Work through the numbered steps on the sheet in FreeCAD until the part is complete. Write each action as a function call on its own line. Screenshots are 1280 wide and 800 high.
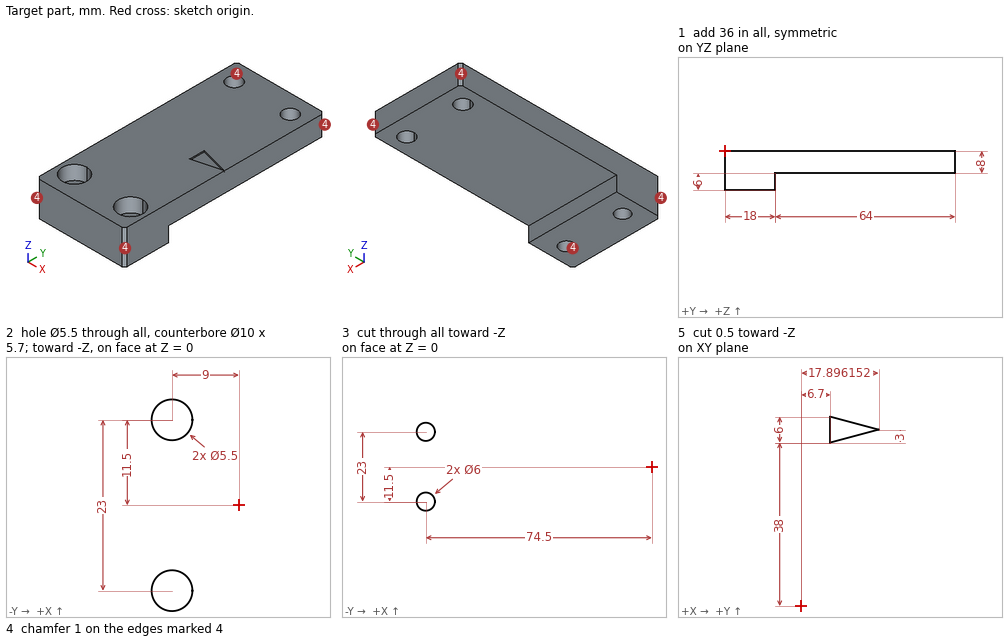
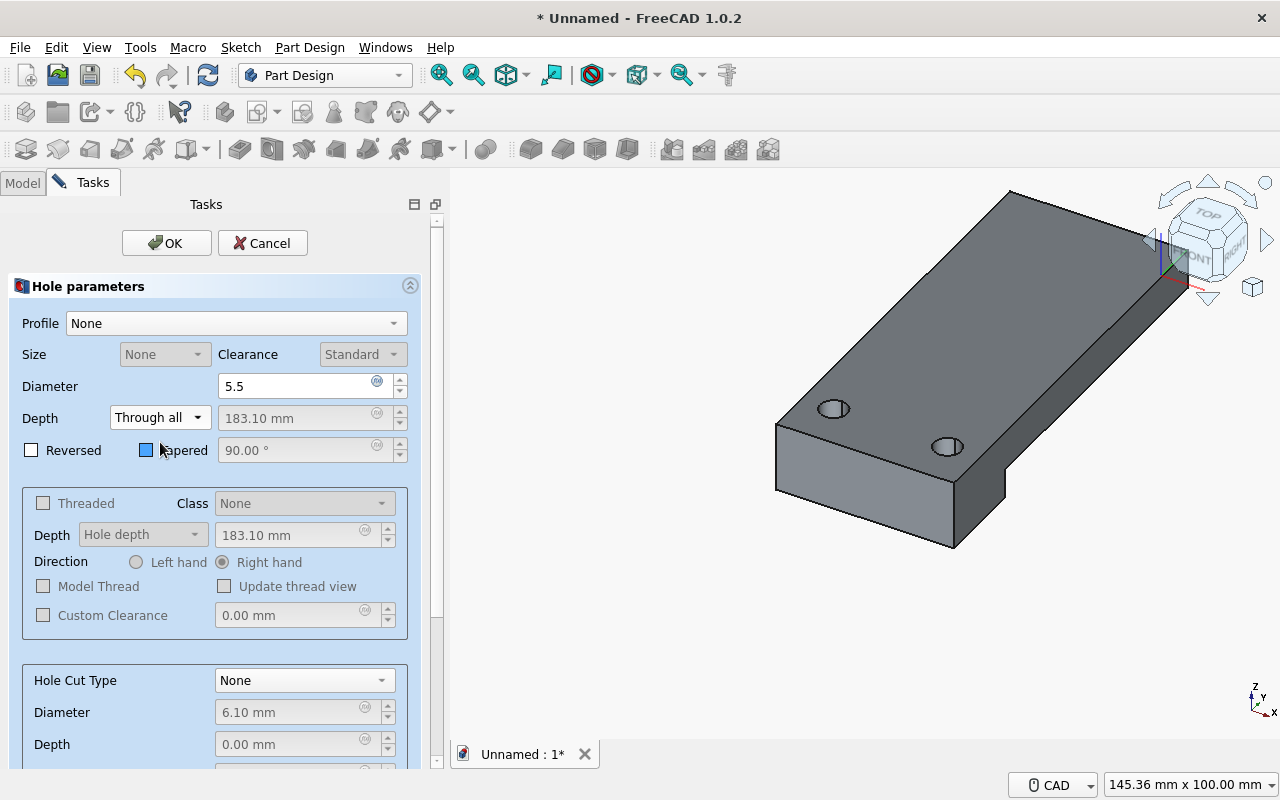
click(306, 680)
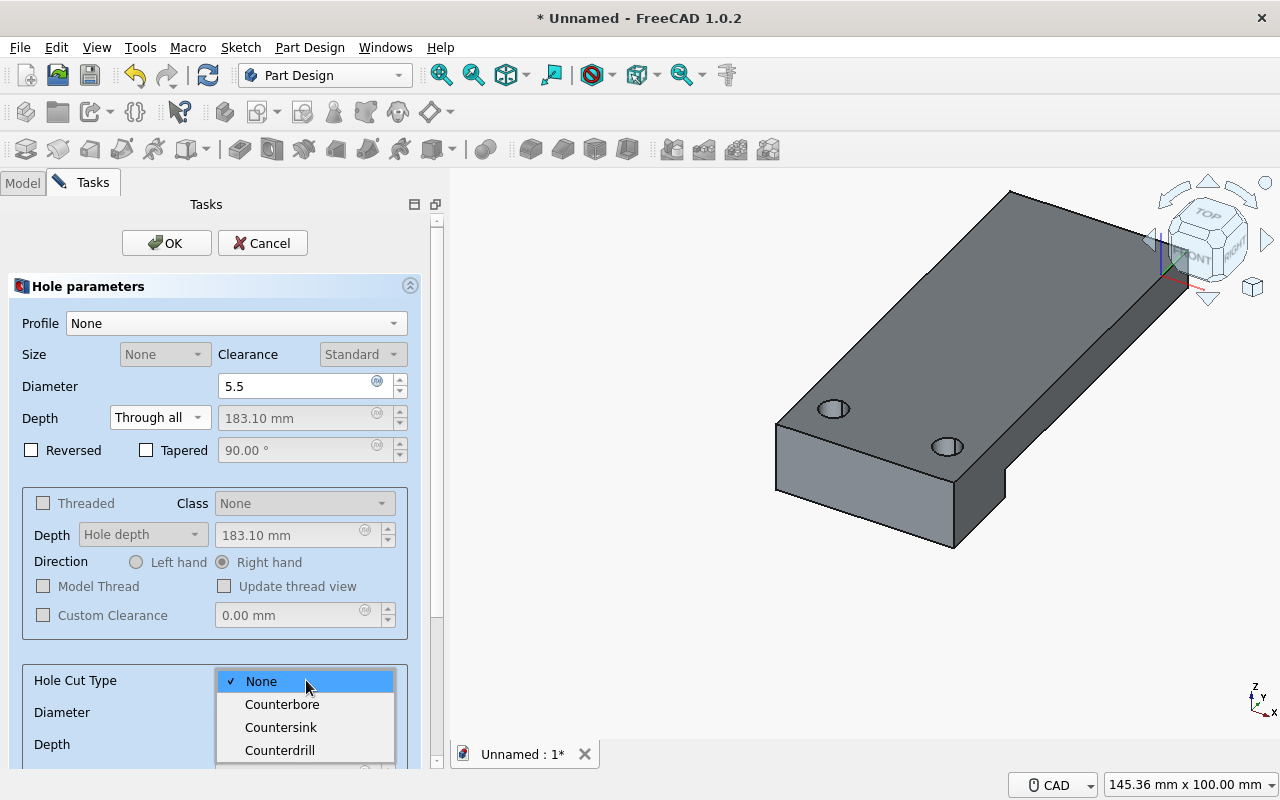
click(304, 704)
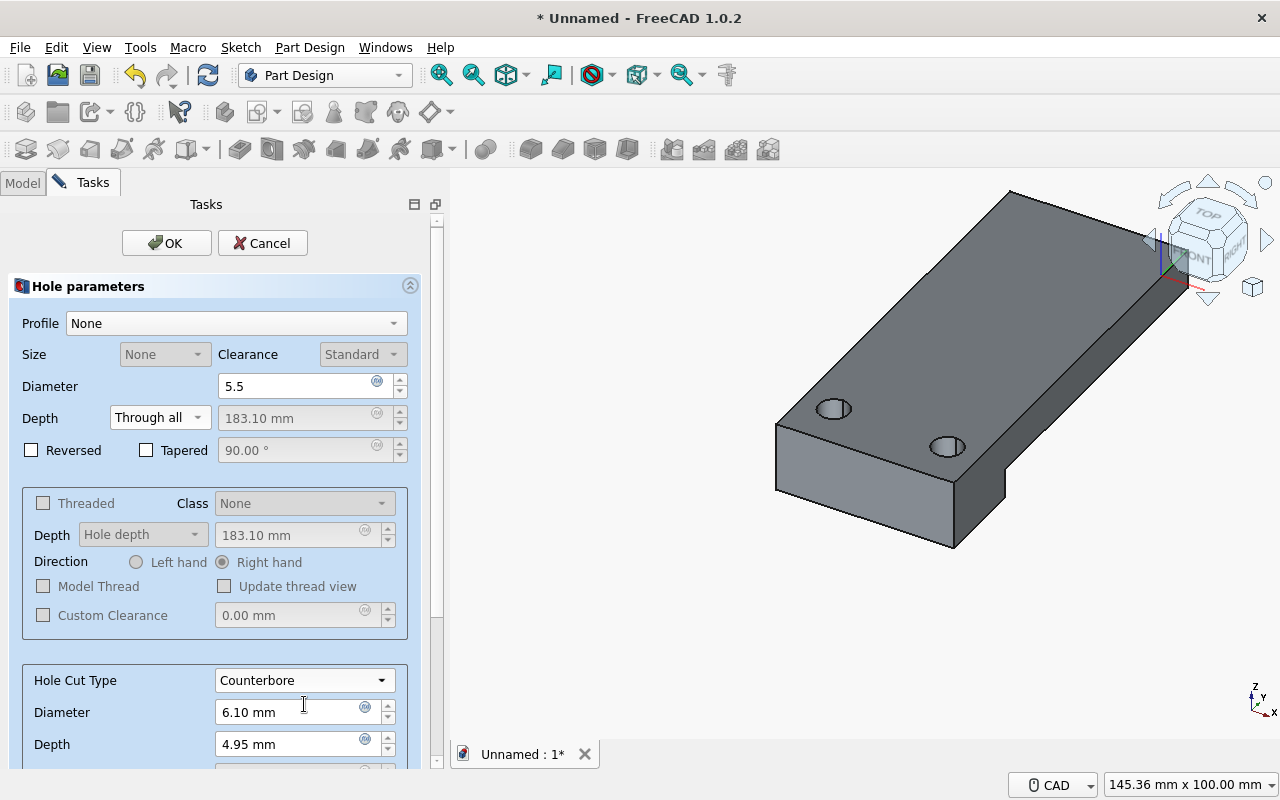
triple_click(298, 712)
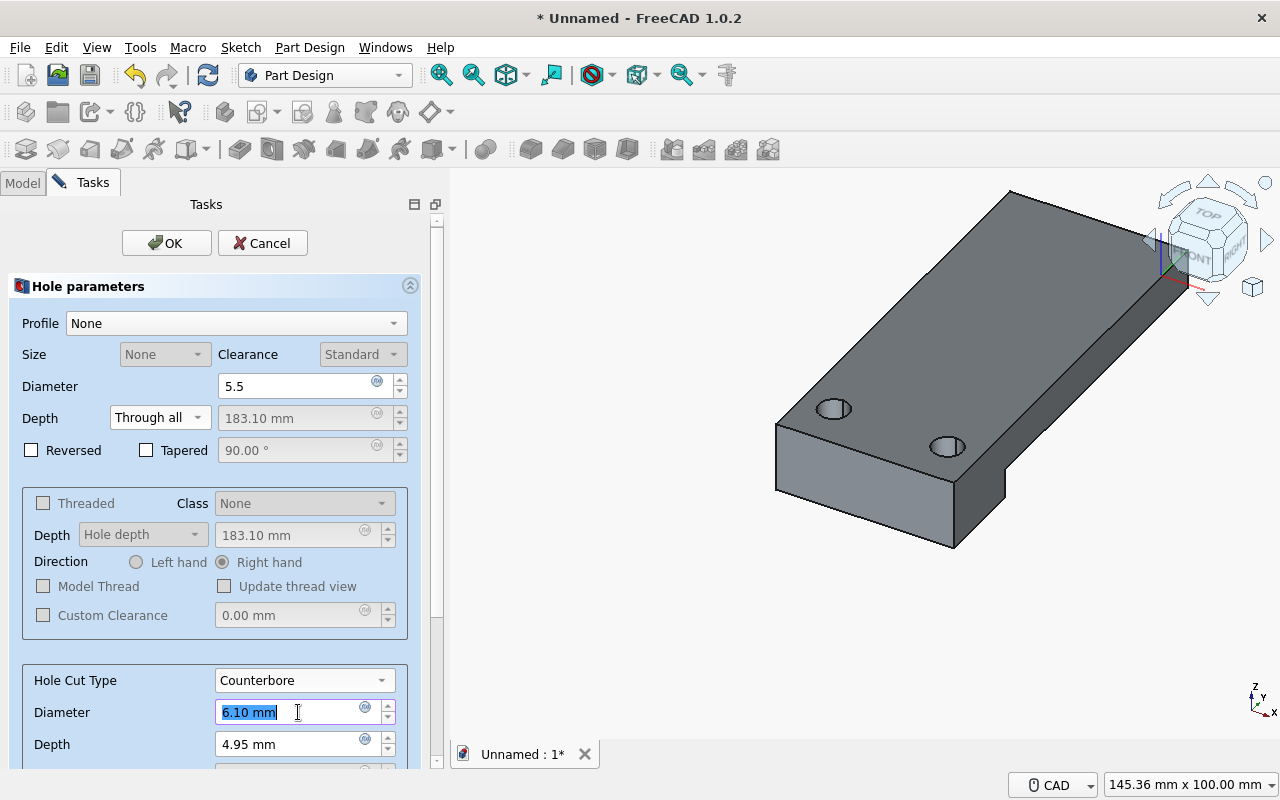
text(10)
key(Tab)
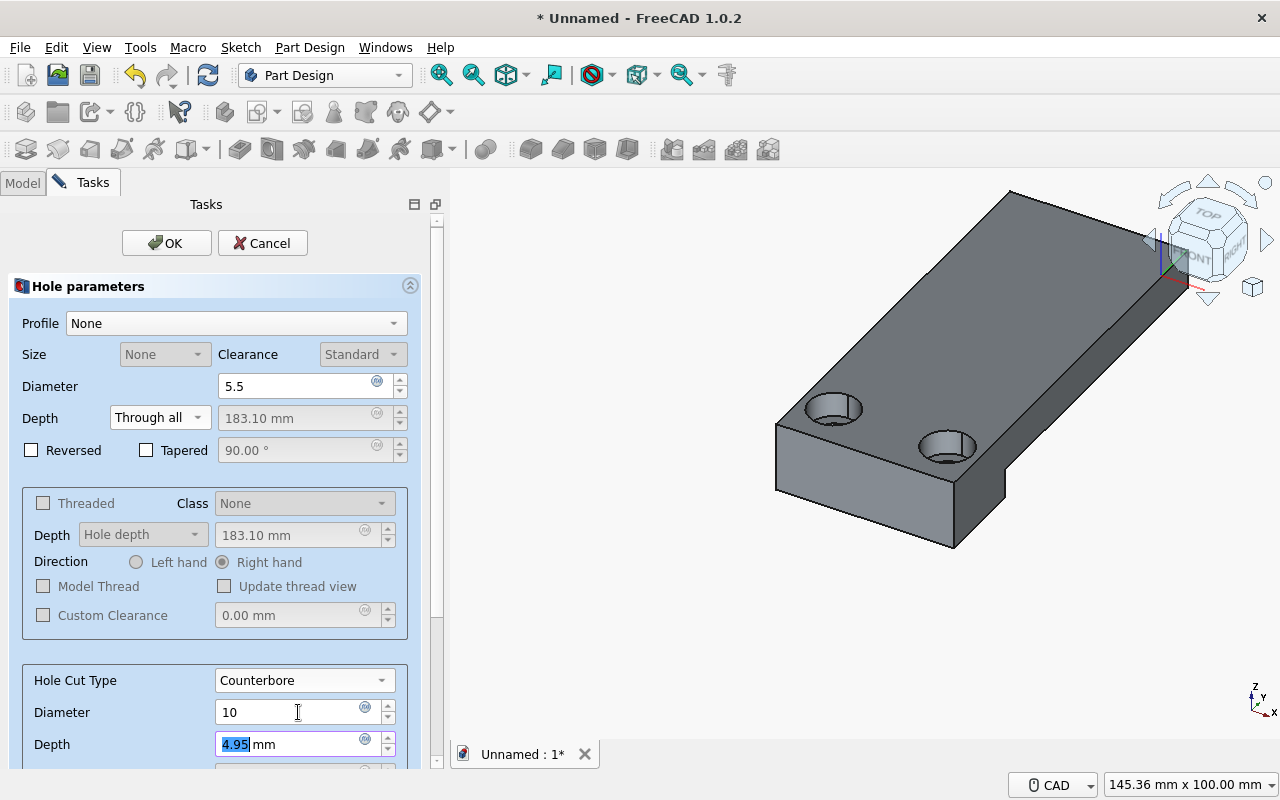
text(5.7)
key(Tab)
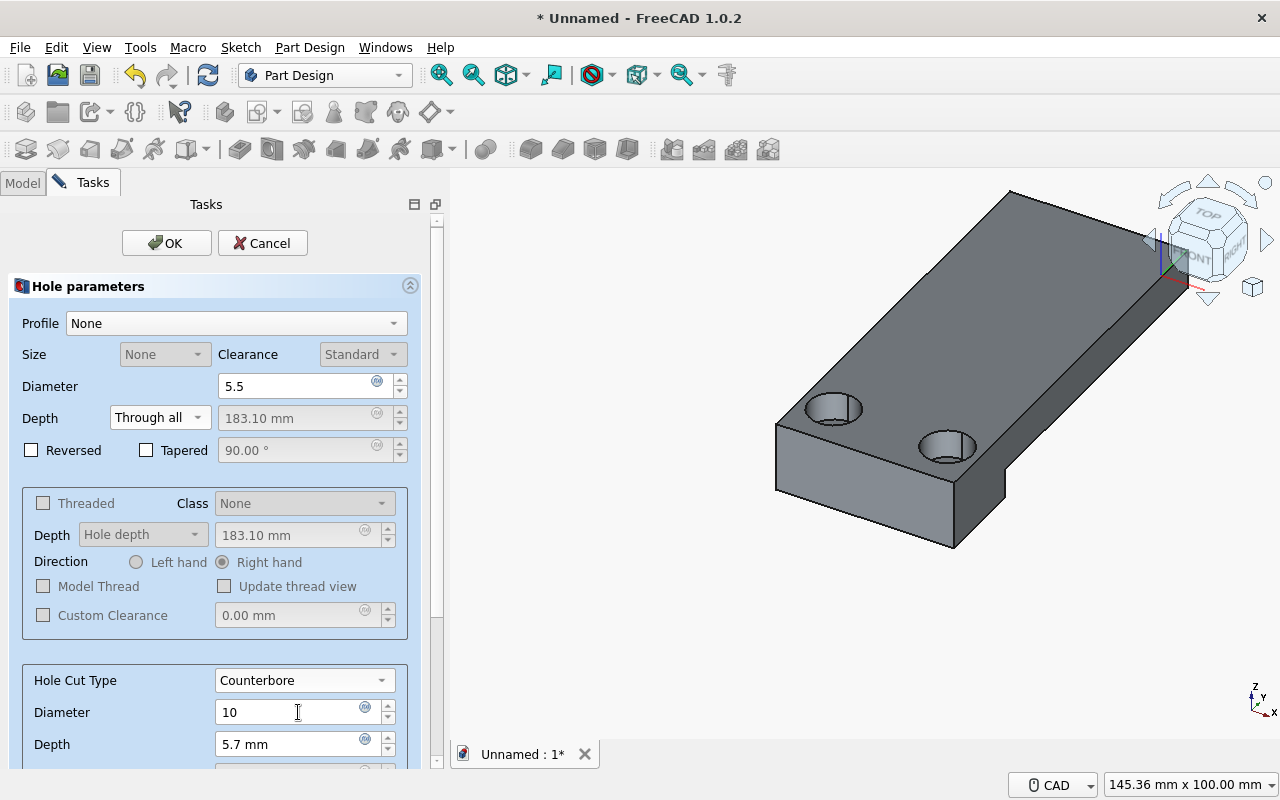
click(167, 243)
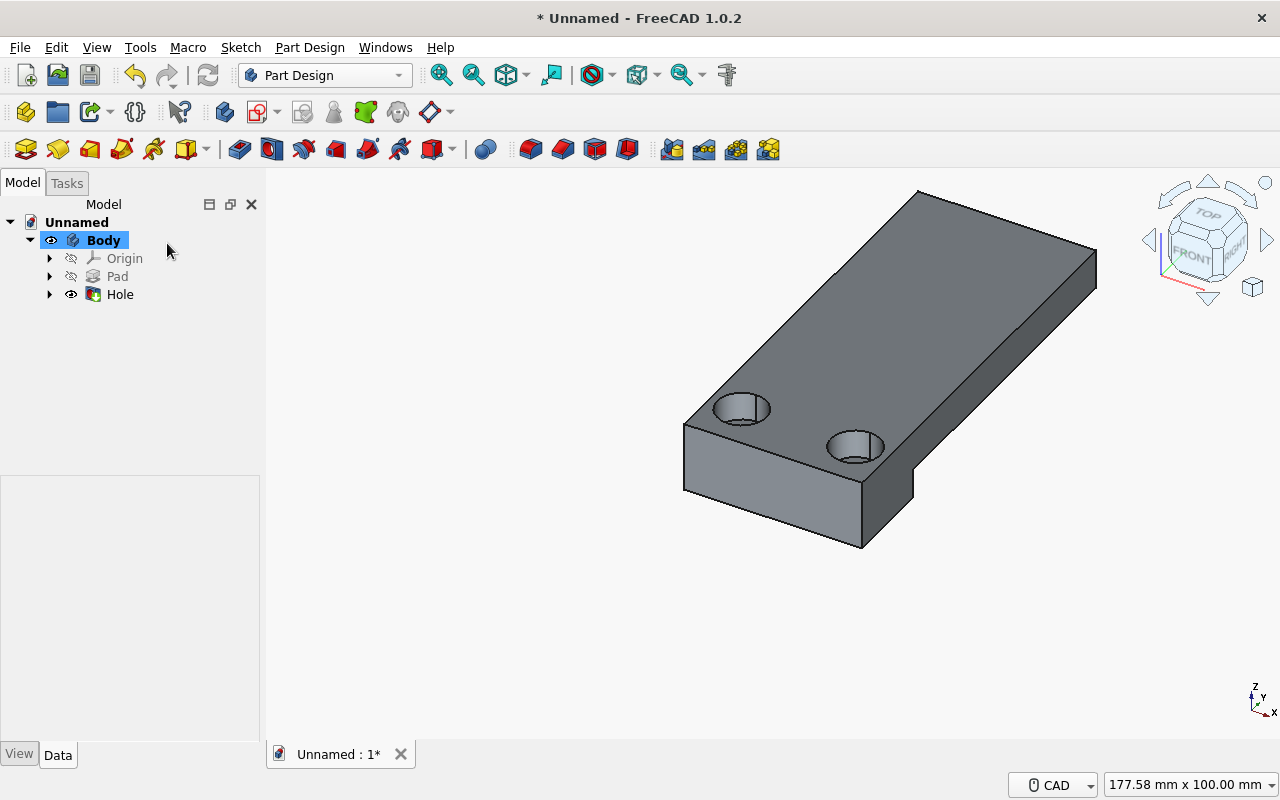
click(923, 303)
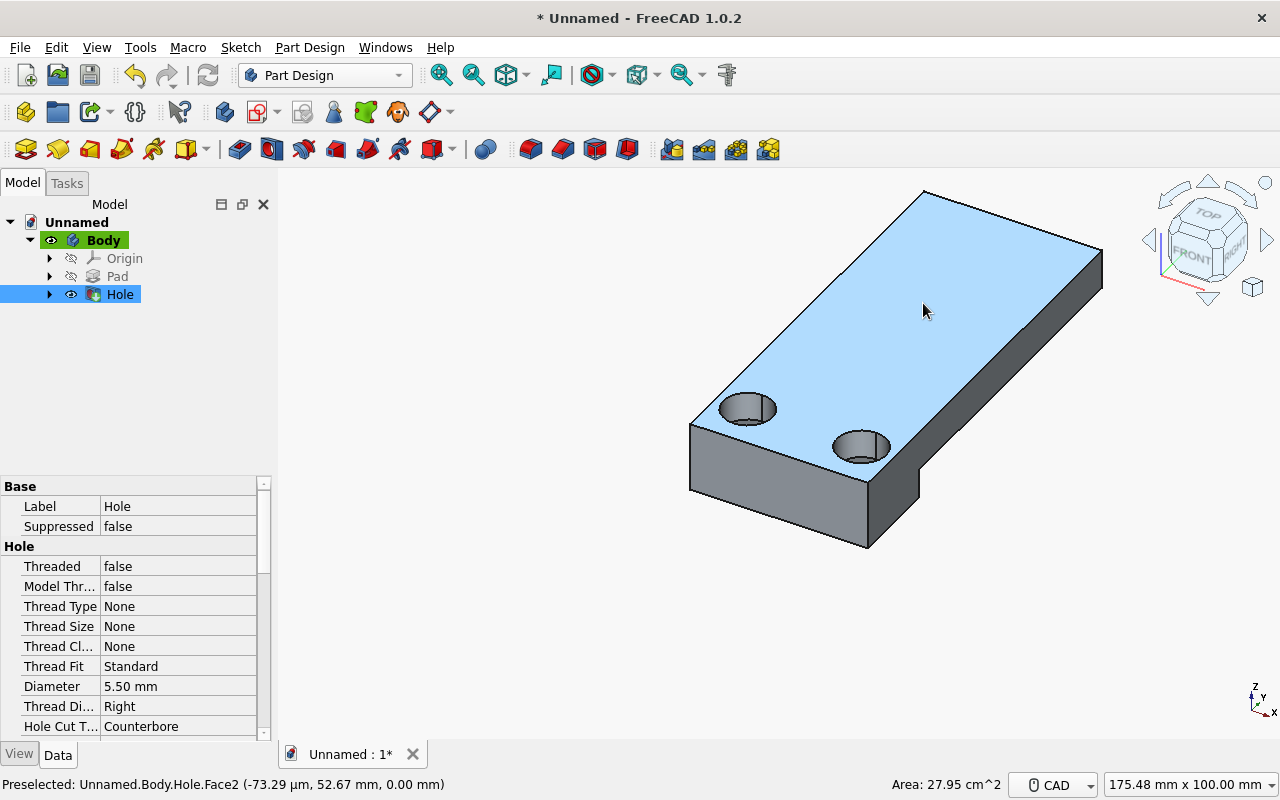
click(258, 112)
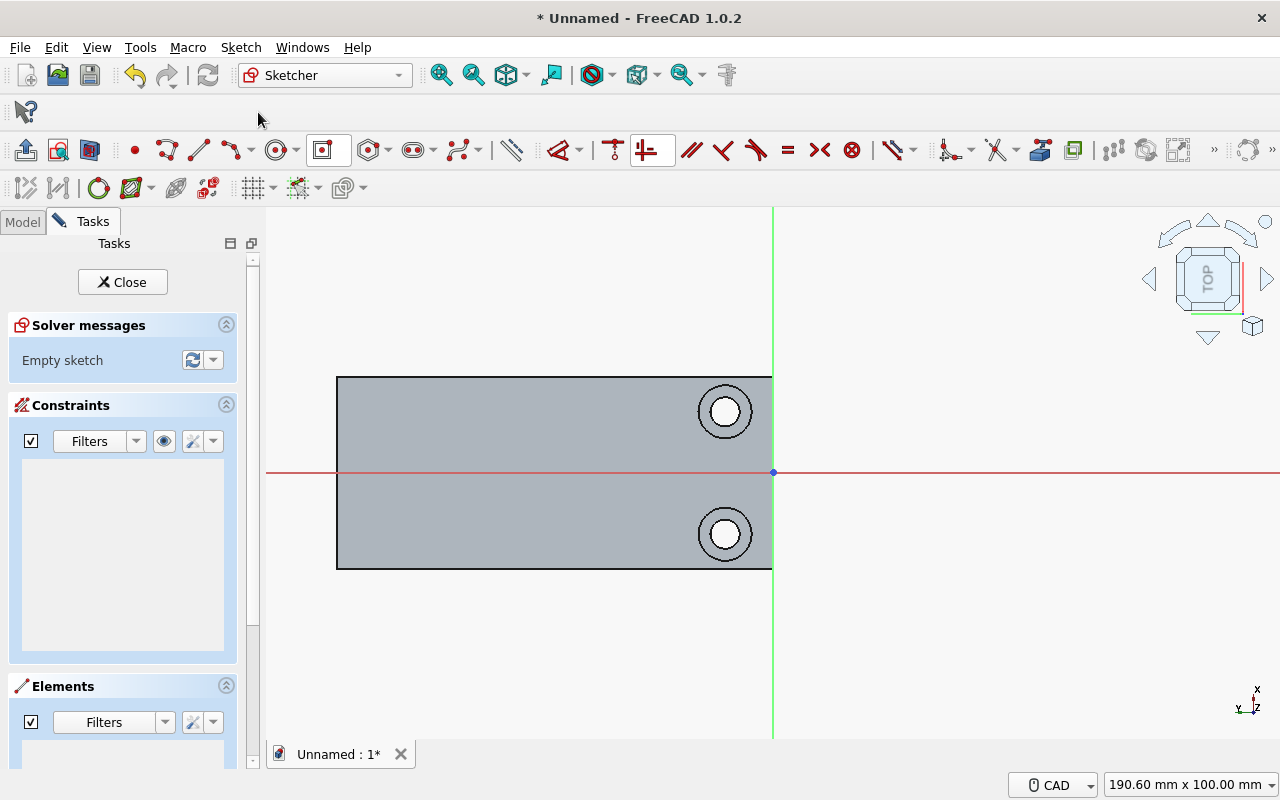
scroll(294, 473, up, 4)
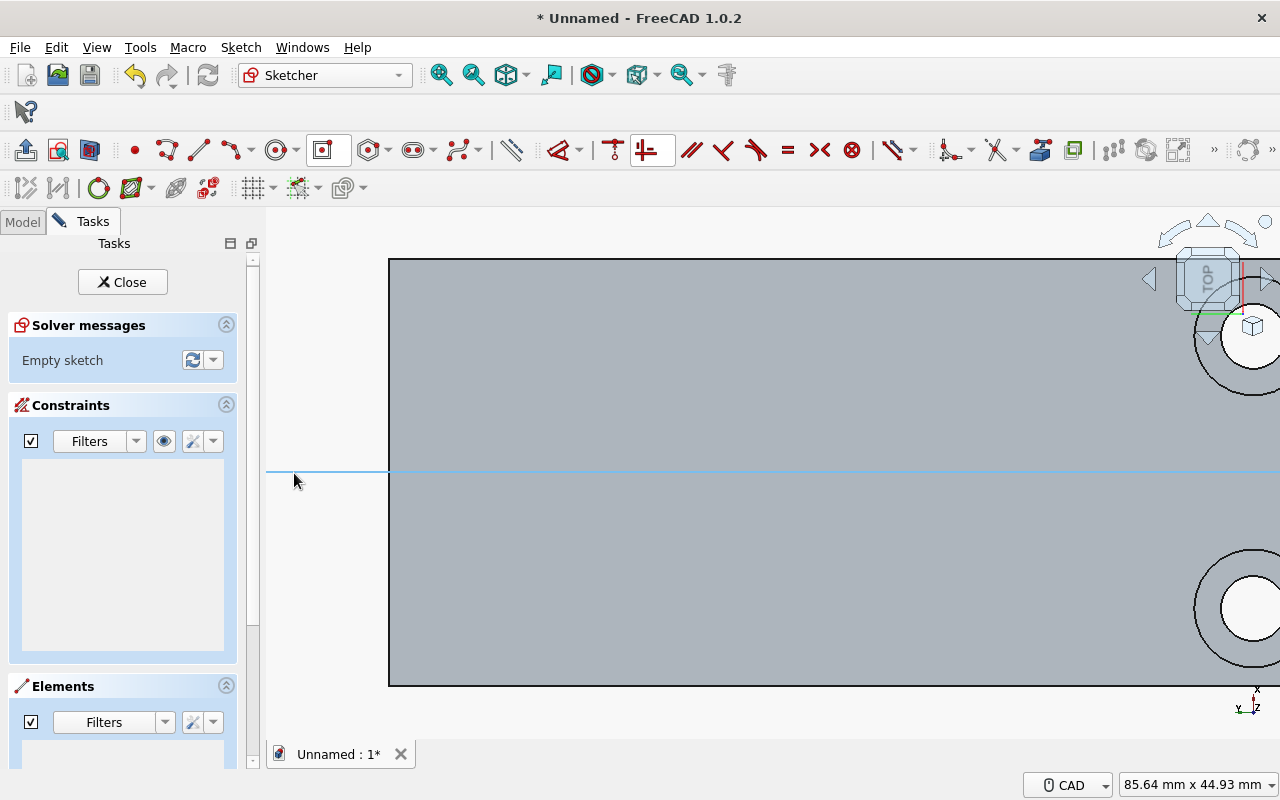
click(276, 150)